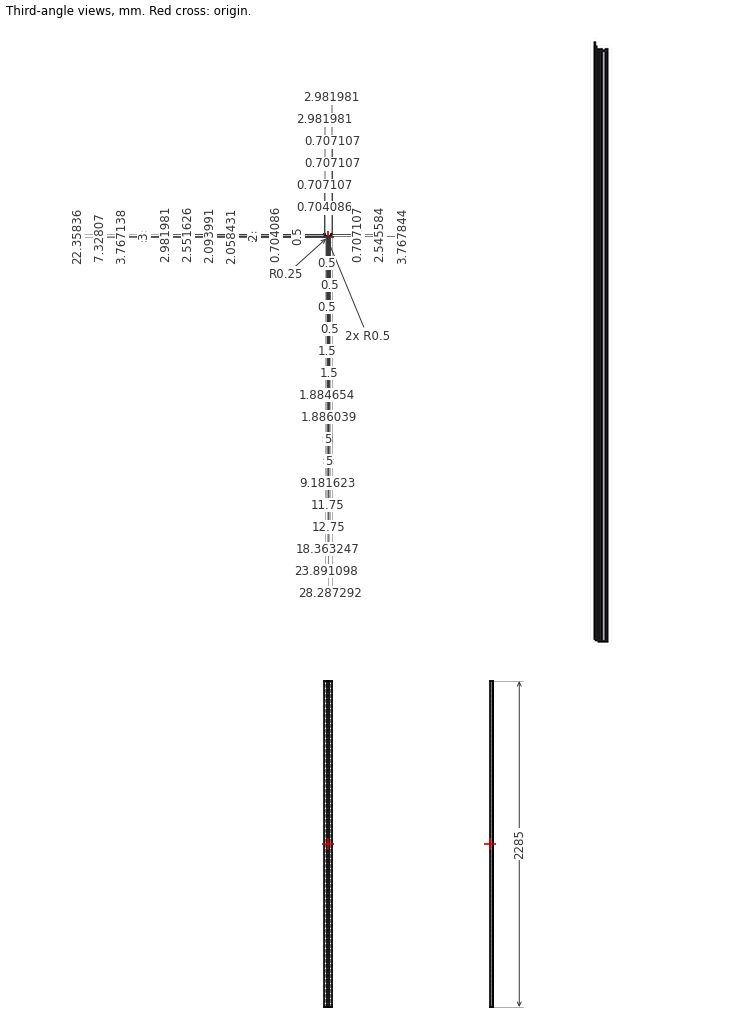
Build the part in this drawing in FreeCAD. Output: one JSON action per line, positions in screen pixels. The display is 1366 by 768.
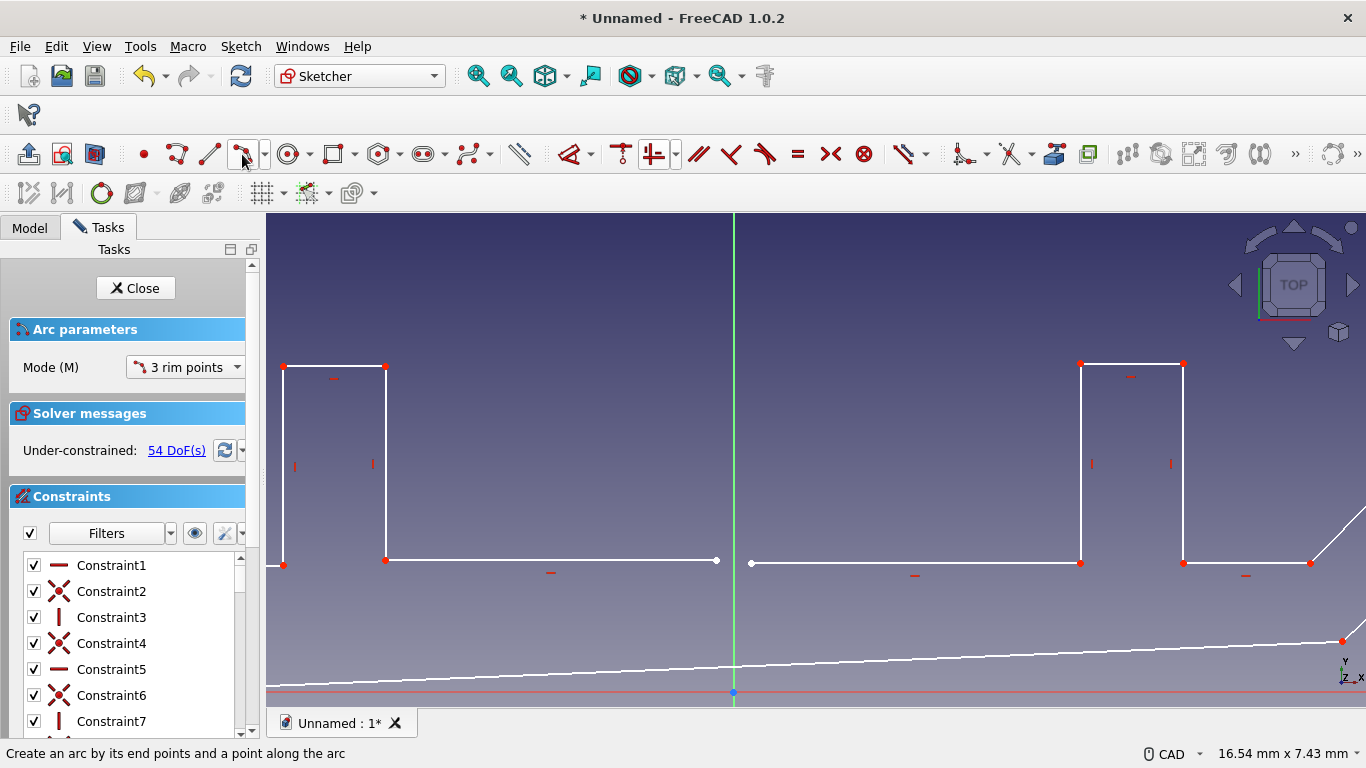
{"action": "scroll", "coordinate": [750, 561], "scroll_direction": "down", "scroll_amount": 9}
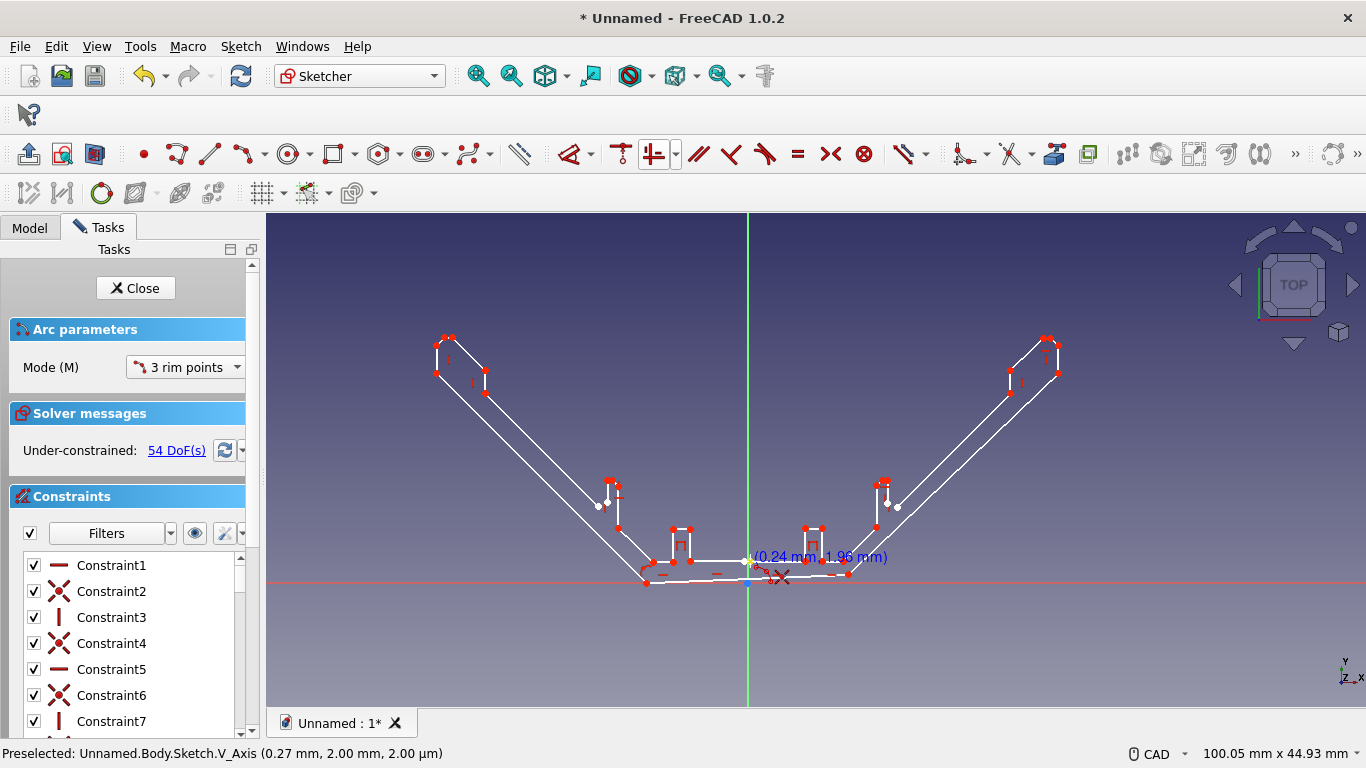
{"action": "scroll", "coordinate": [608, 503], "scroll_direction": "up", "scroll_amount": 3}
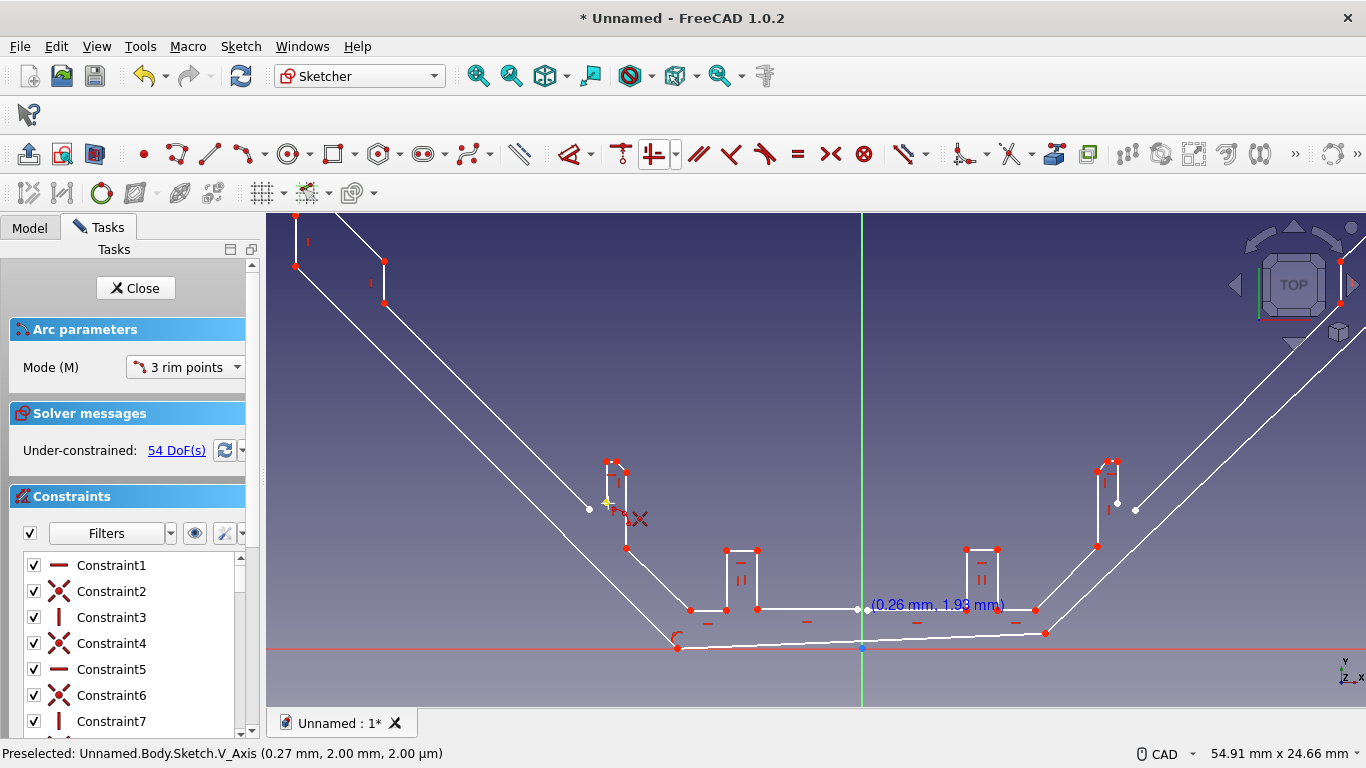
{"action": "left_click", "coordinate": [607, 502]}
{"action": "left_click", "coordinate": [590, 509]}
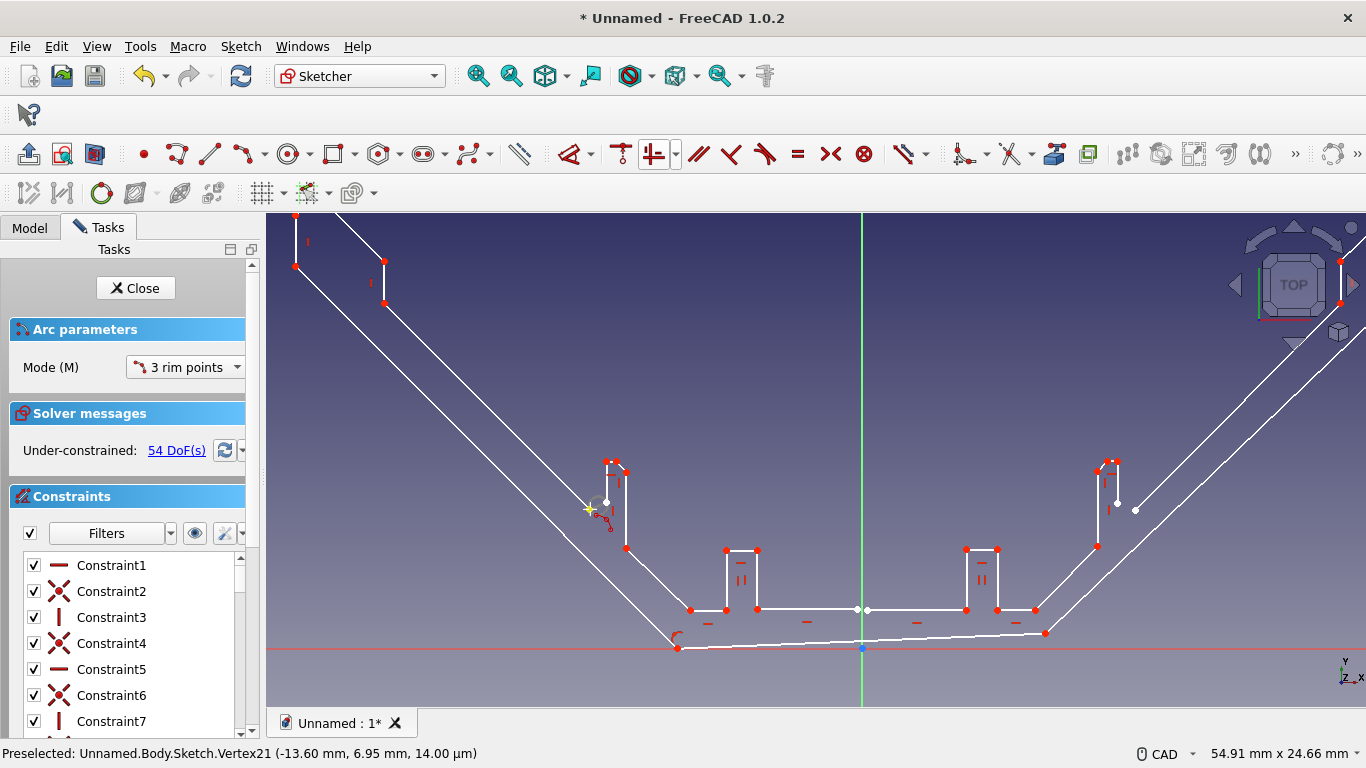
{"action": "scroll", "coordinate": [601, 511], "scroll_direction": "up", "scroll_amount": 5}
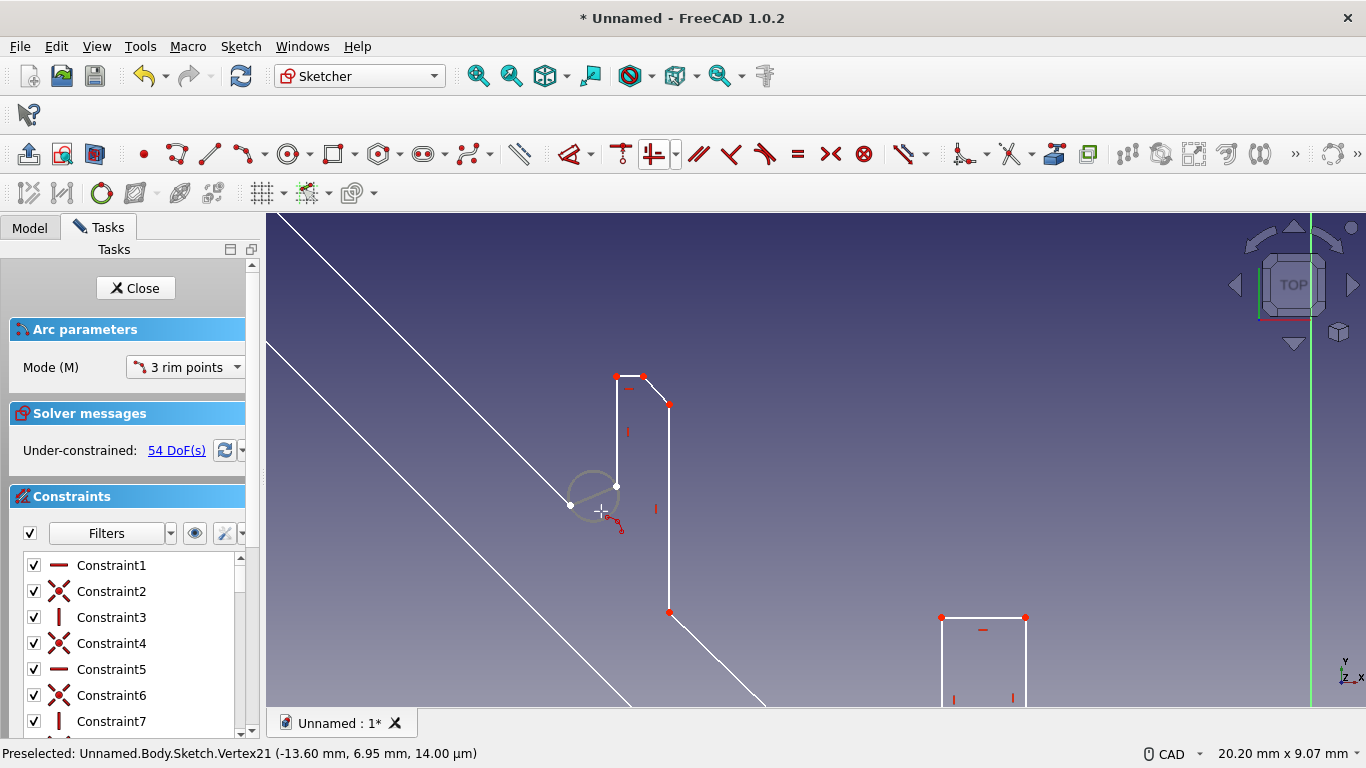
{"action": "left_click", "coordinate": [600, 511]}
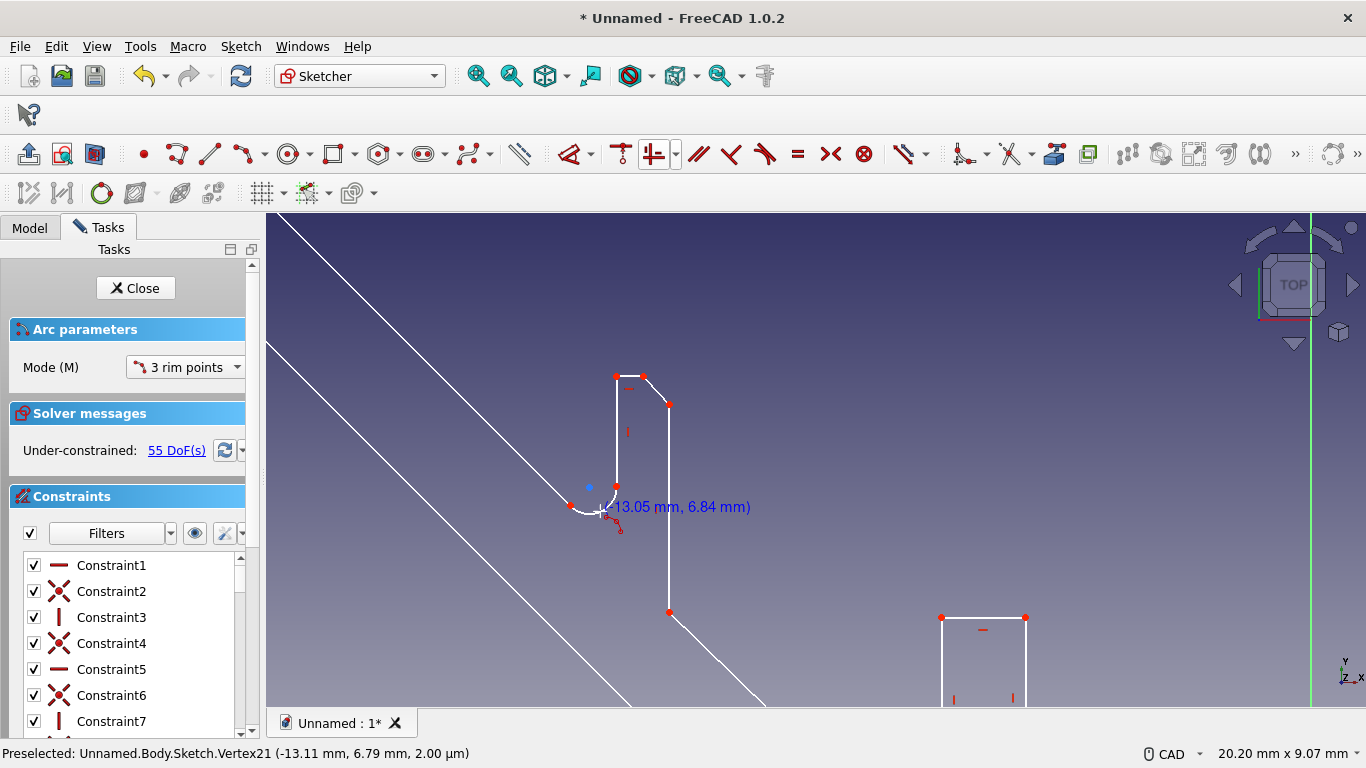
{"action": "scroll", "coordinate": [605, 507], "scroll_direction": "down", "scroll_amount": 8}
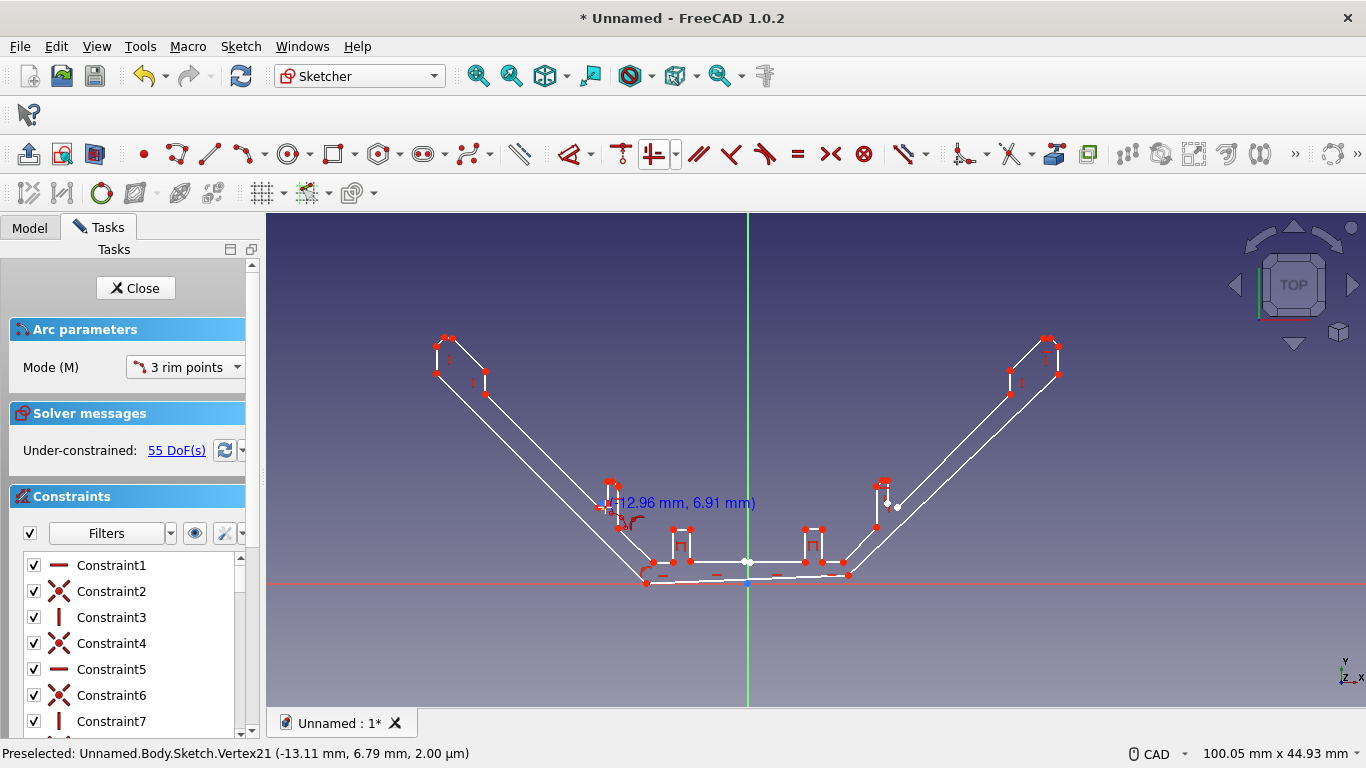
{"action": "scroll", "coordinate": [897, 507], "scroll_direction": "up", "scroll_amount": 3}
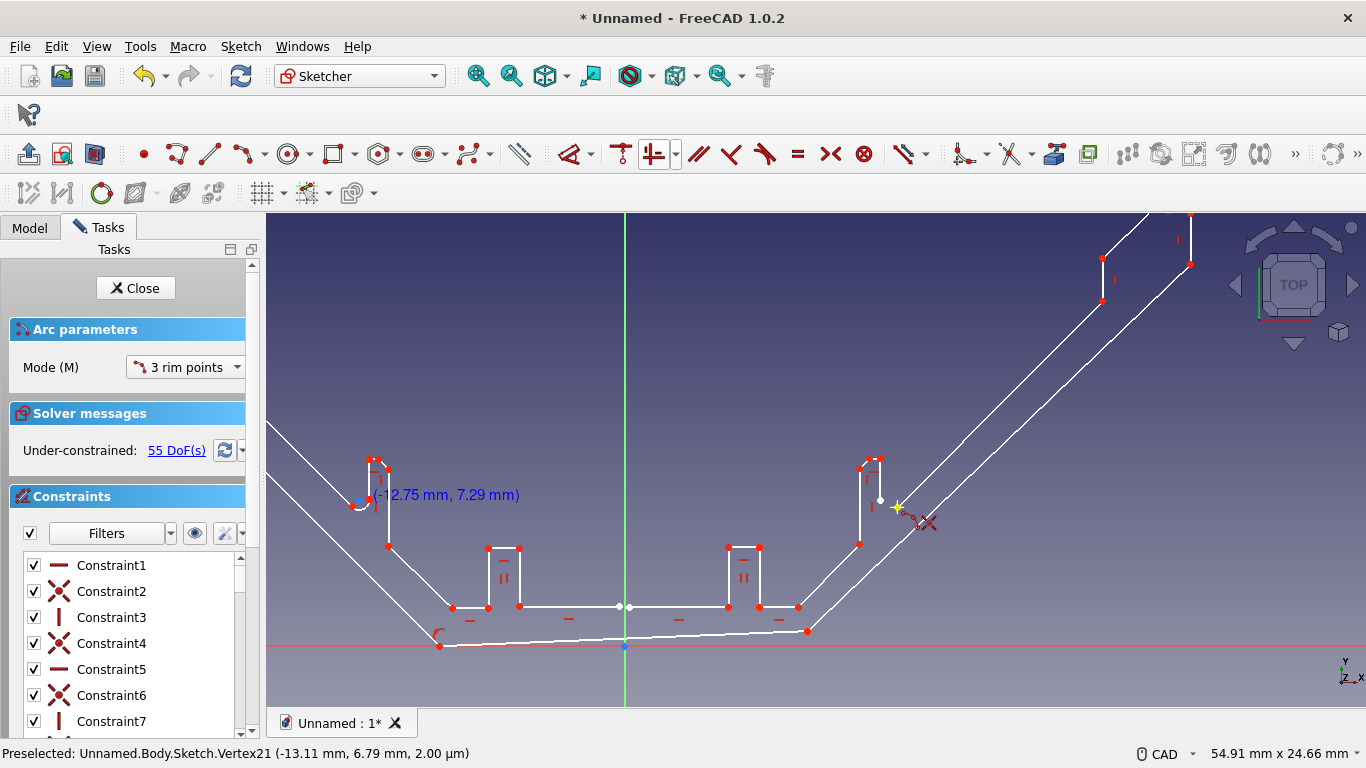
{"action": "left_click", "coordinate": [898, 508]}
{"action": "left_click", "coordinate": [880, 501]}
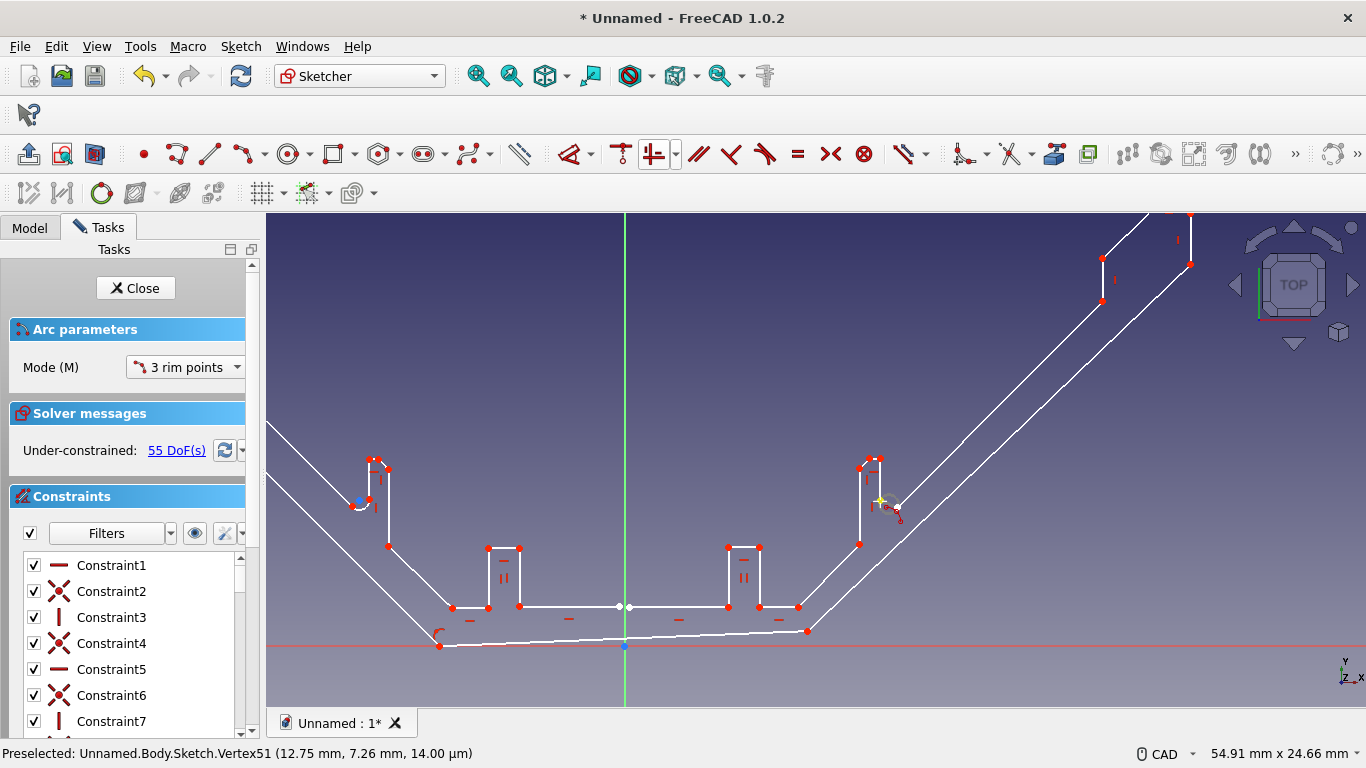
{"action": "scroll", "coordinate": [886, 509], "scroll_direction": "up", "scroll_amount": 5}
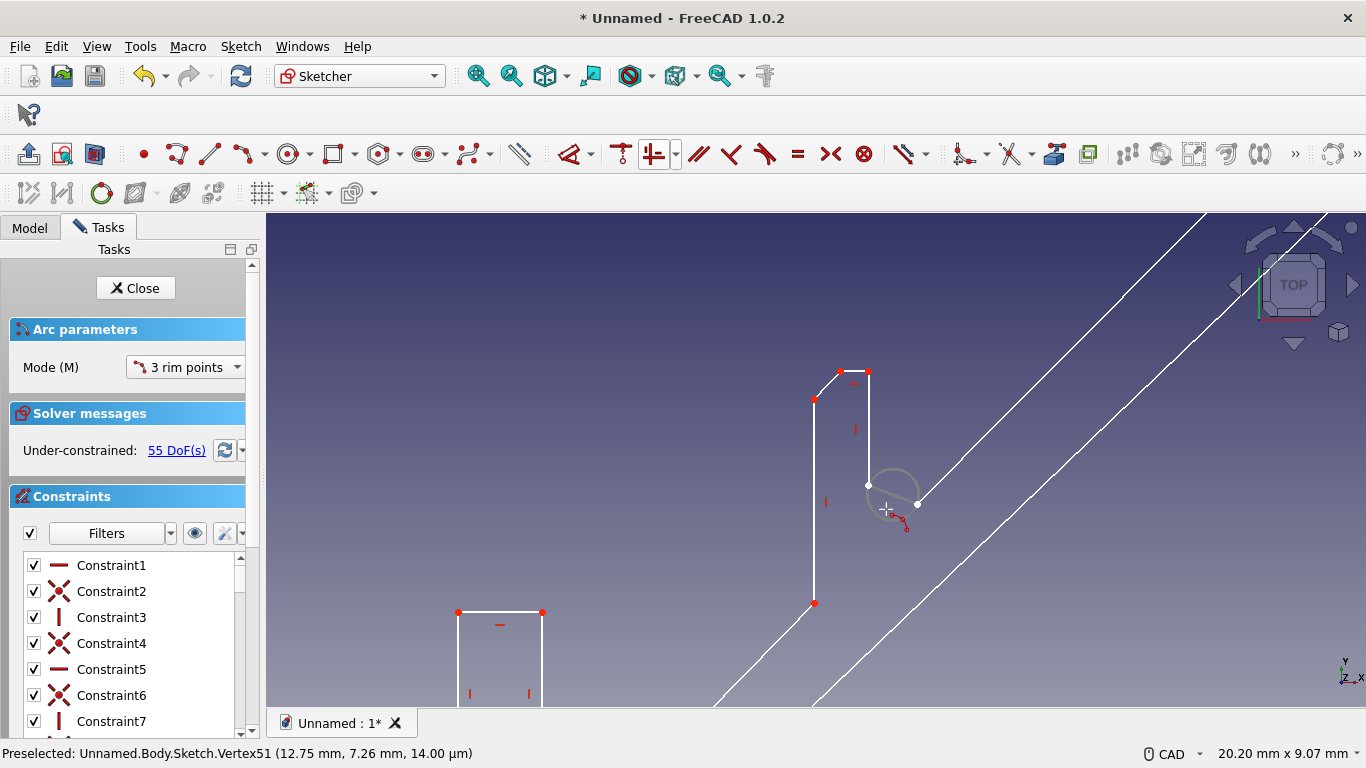
{"action": "left_click", "coordinate": [885, 507]}